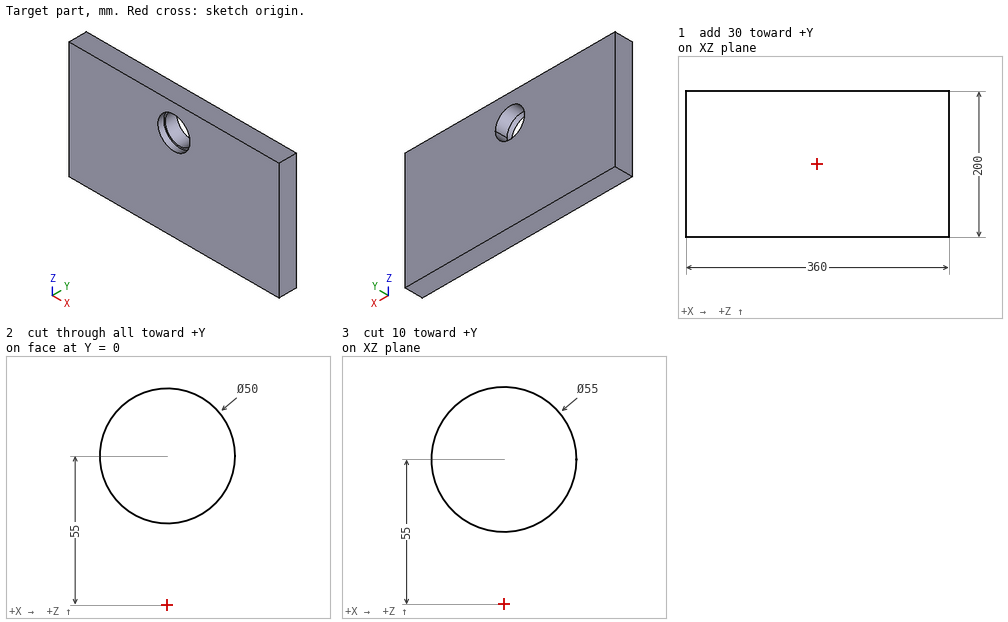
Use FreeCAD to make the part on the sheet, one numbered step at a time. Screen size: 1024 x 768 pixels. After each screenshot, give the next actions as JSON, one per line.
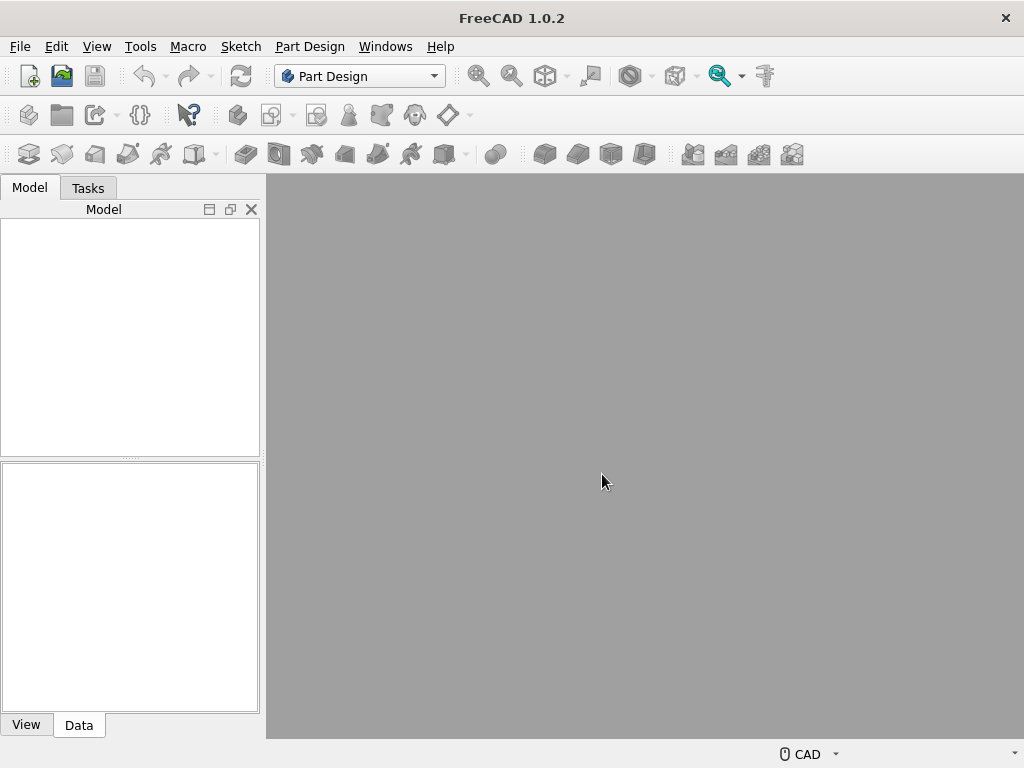
{"action": "key", "text": "ctrl+n"}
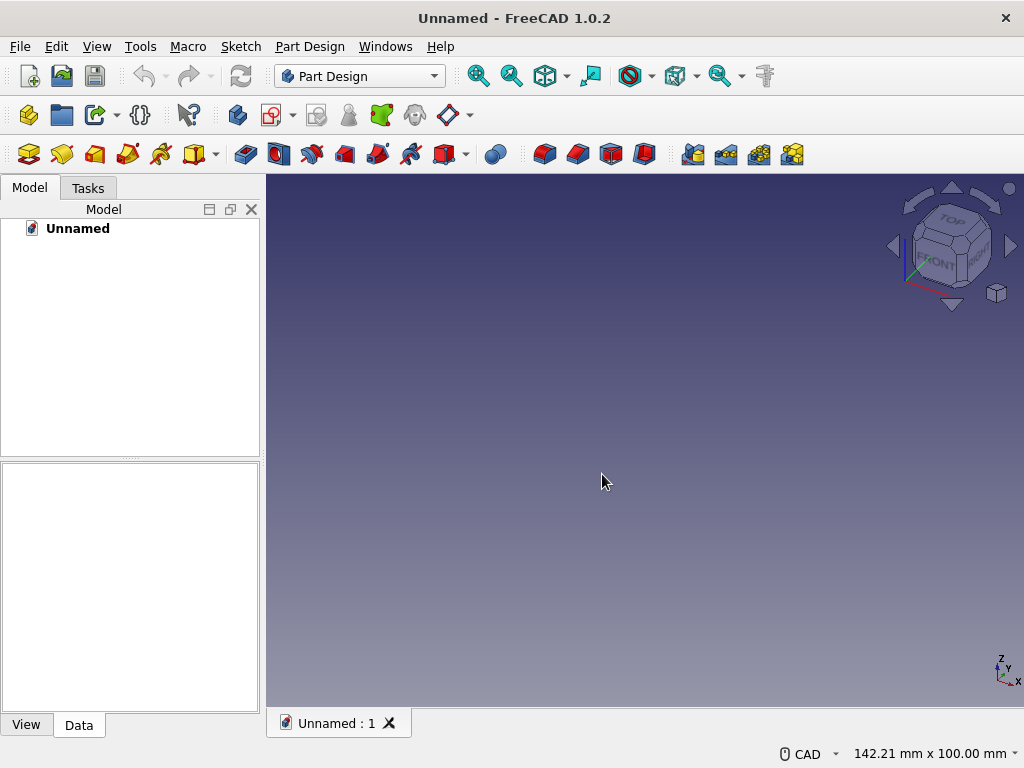
{"action": "left_click", "coordinate": [270, 116]}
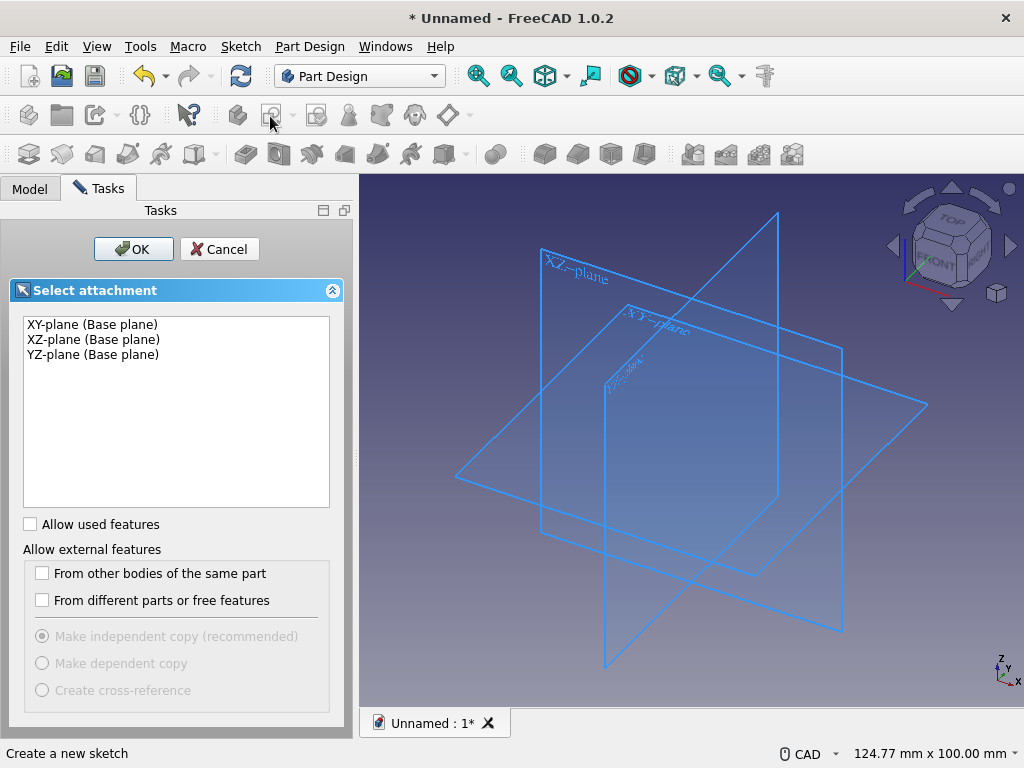
{"action": "left_click", "coordinate": [84, 340]}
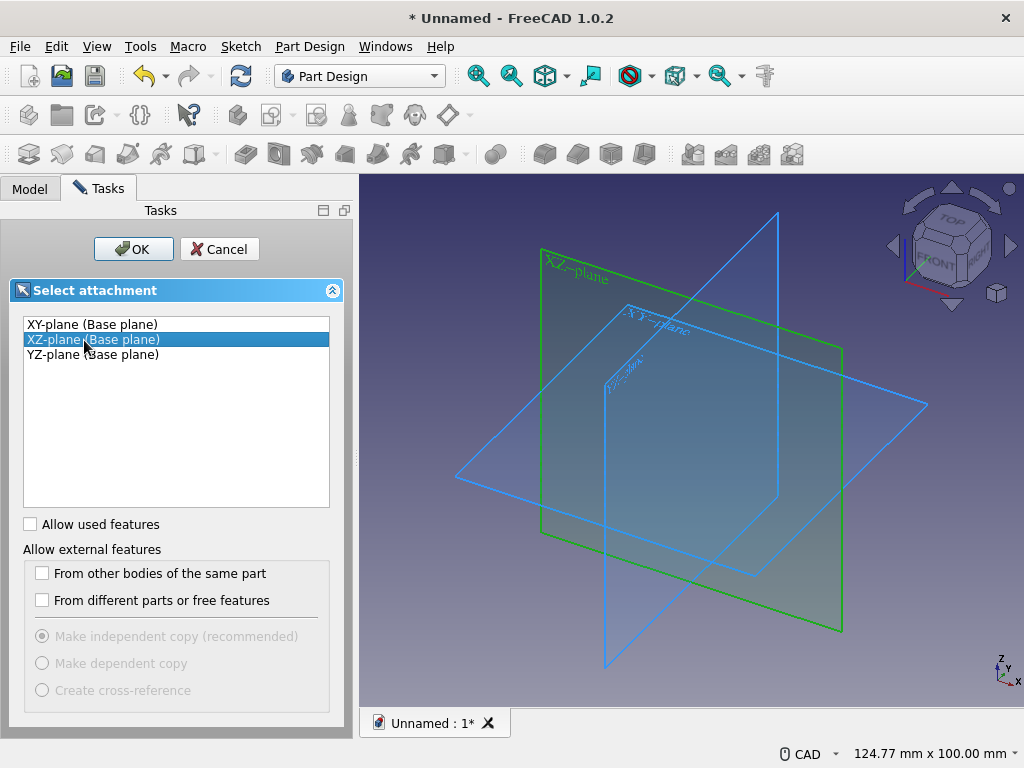
{"action": "left_click", "coordinate": [134, 249]}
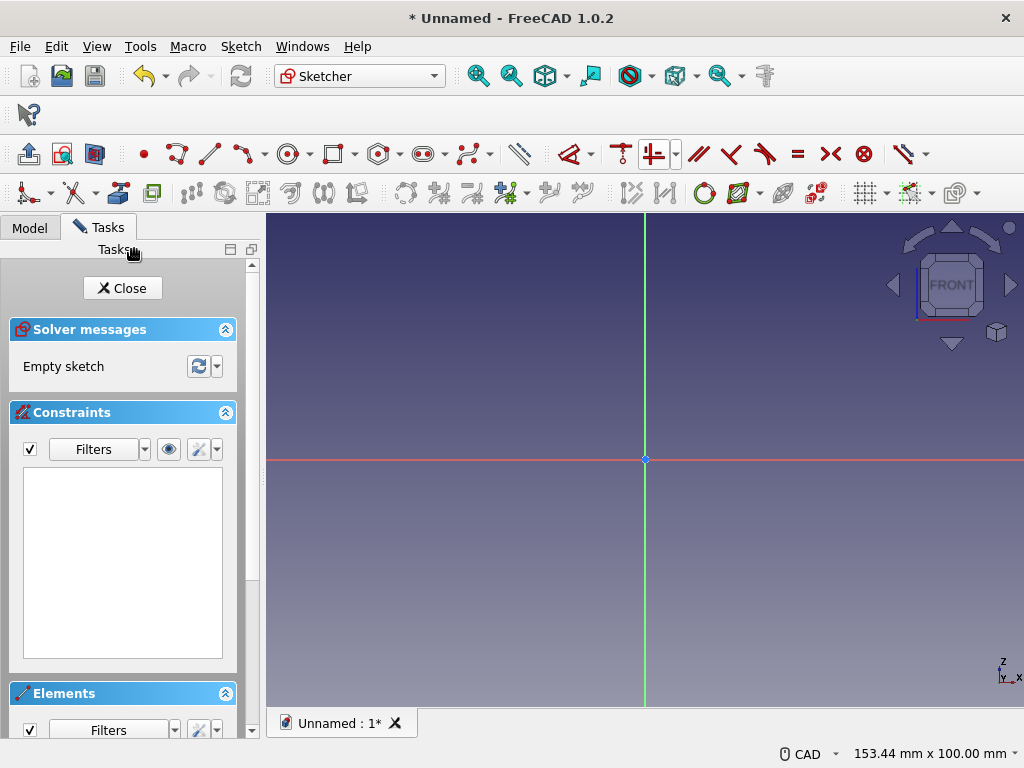
{"action": "scroll", "coordinate": [554, 460], "scroll_direction": "down", "scroll_amount": 7}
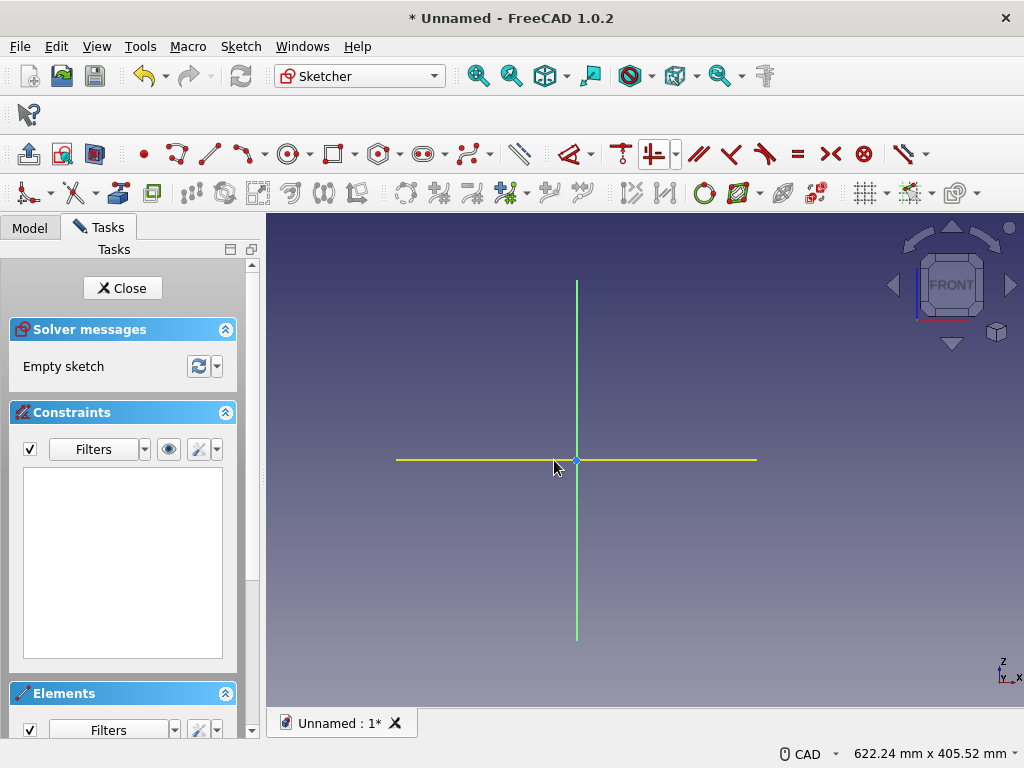
{"action": "key", "text": "g v"}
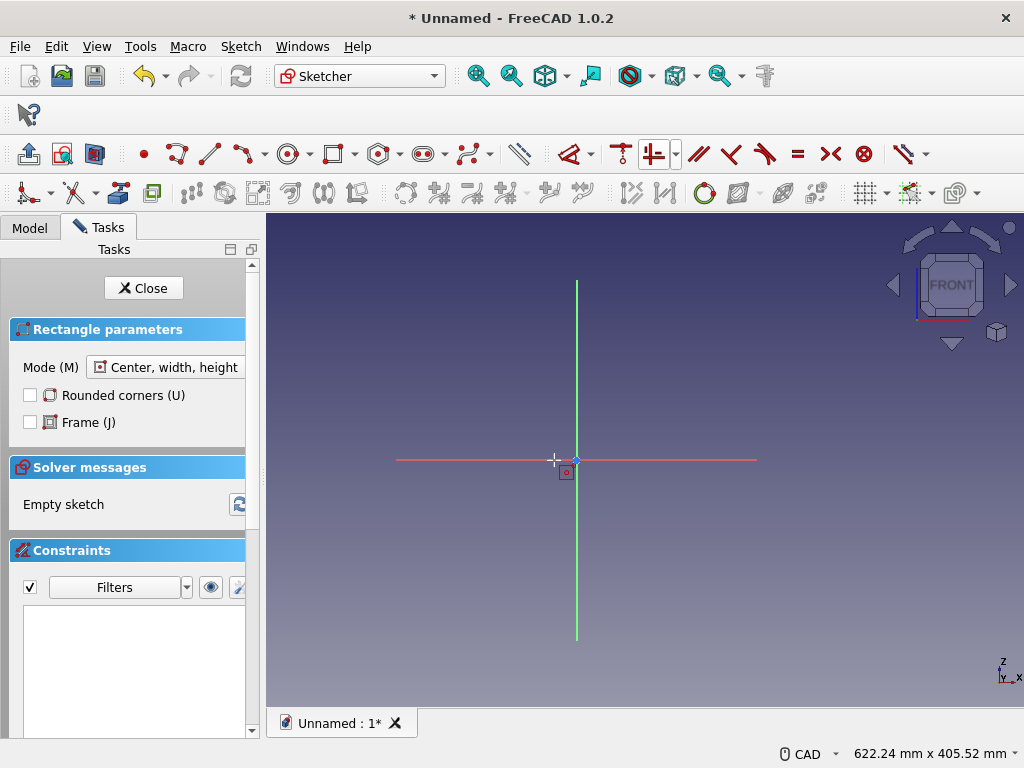
{"action": "left_click", "coordinate": [577, 460]}
{"action": "left_click", "coordinate": [796, 339]}
{"action": "key", "text": "Escape"}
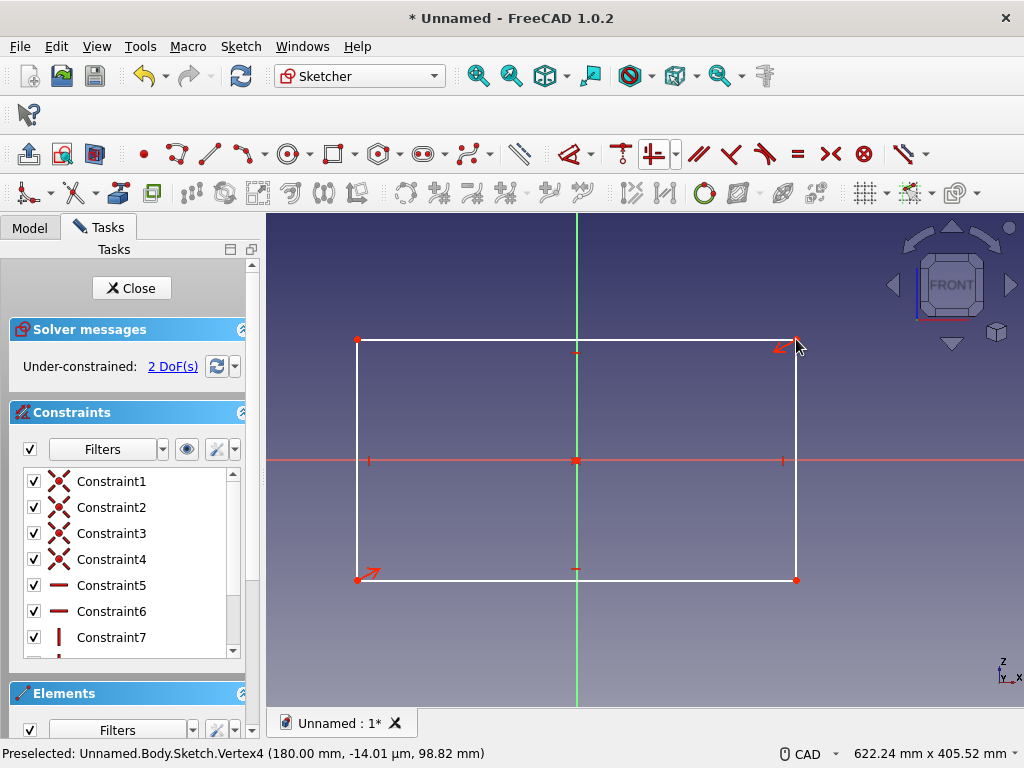
{"action": "left_click", "coordinate": [489, 581]}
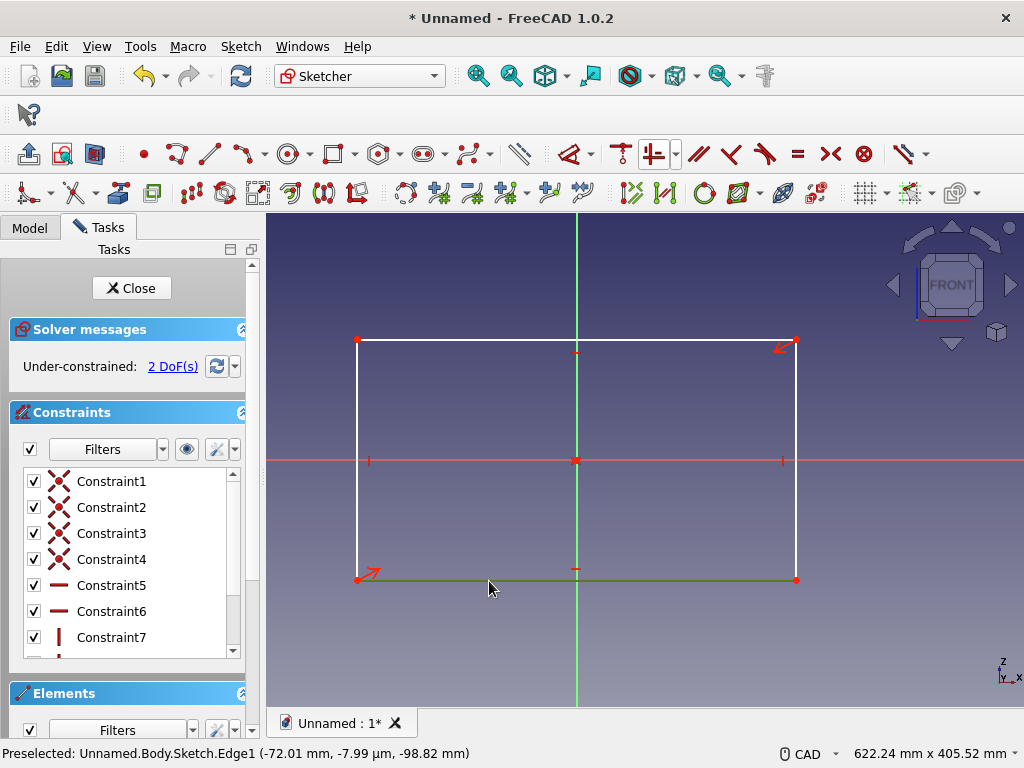
{"action": "key", "text": "l"}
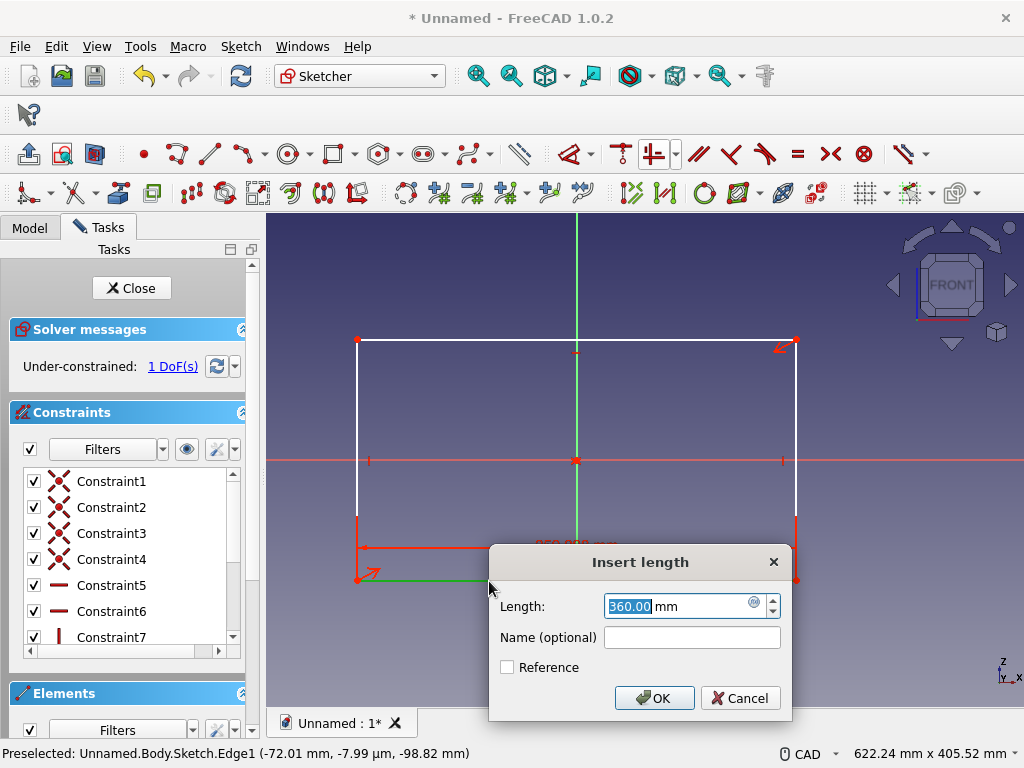
{"action": "type", "text": "360"}
{"action": "key", "text": "Return"}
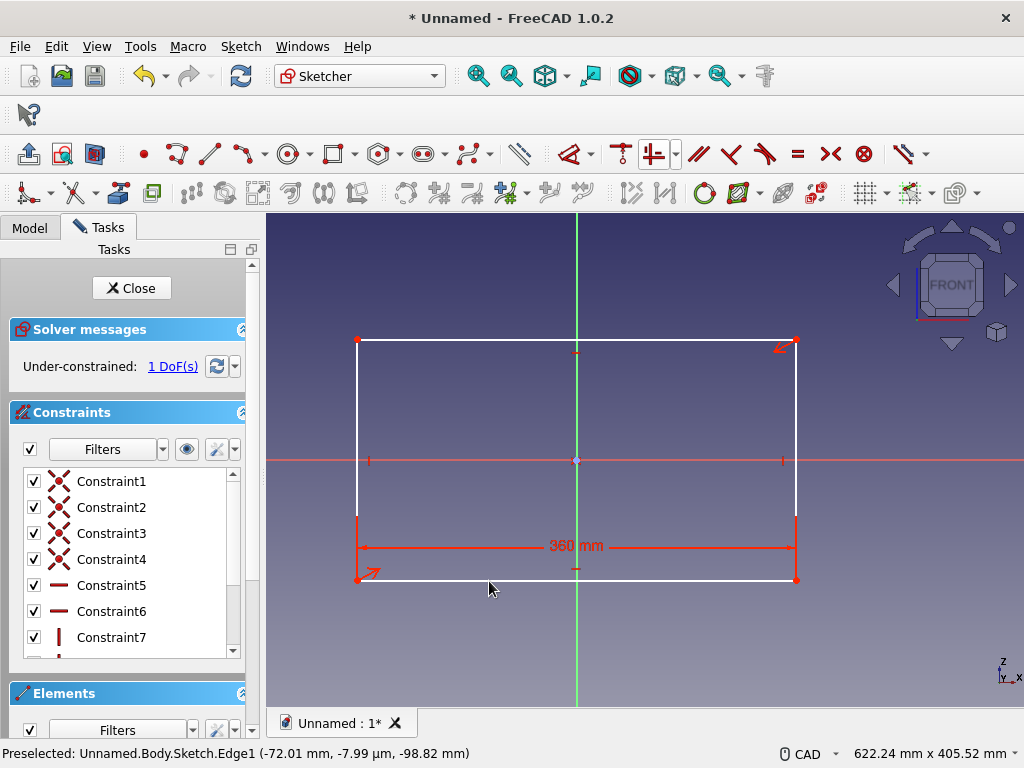
{"action": "left_click", "coordinate": [796, 509]}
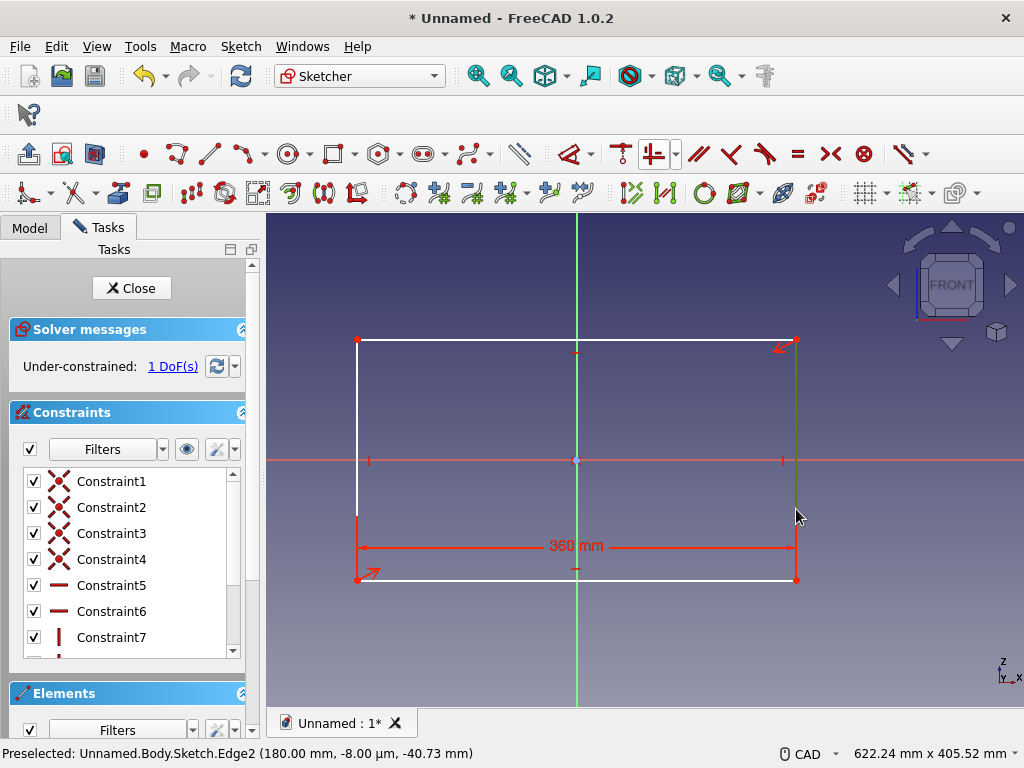
{"action": "left_click", "coordinate": [590, 154]}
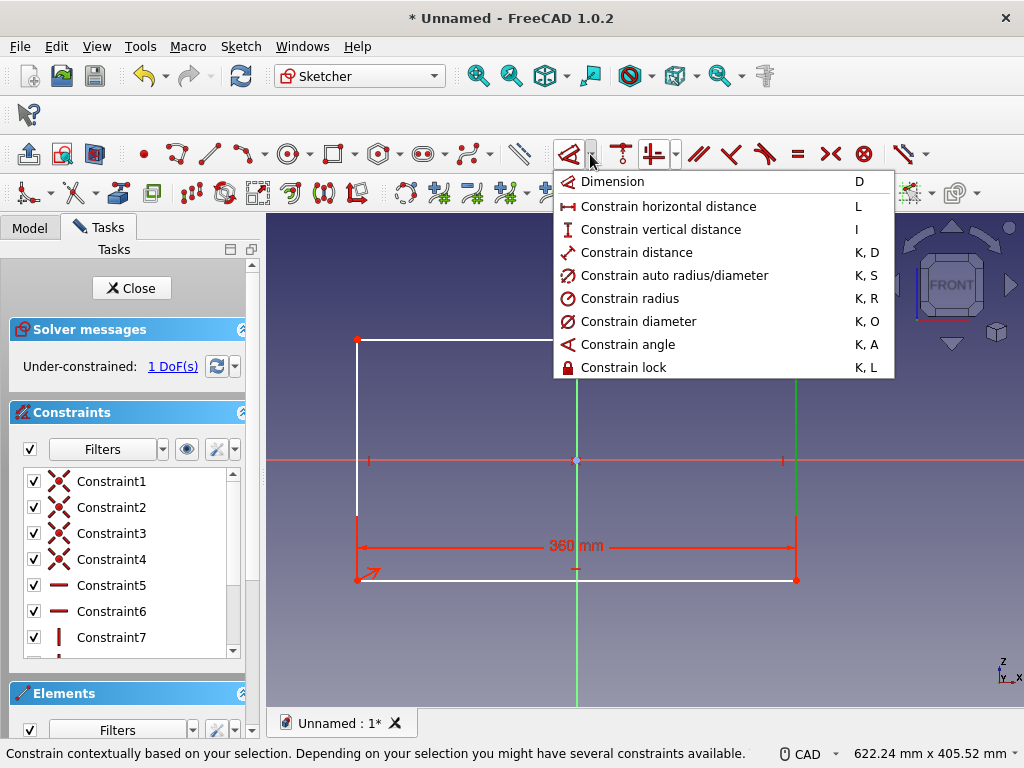
{"action": "left_click", "coordinate": [724, 230]}